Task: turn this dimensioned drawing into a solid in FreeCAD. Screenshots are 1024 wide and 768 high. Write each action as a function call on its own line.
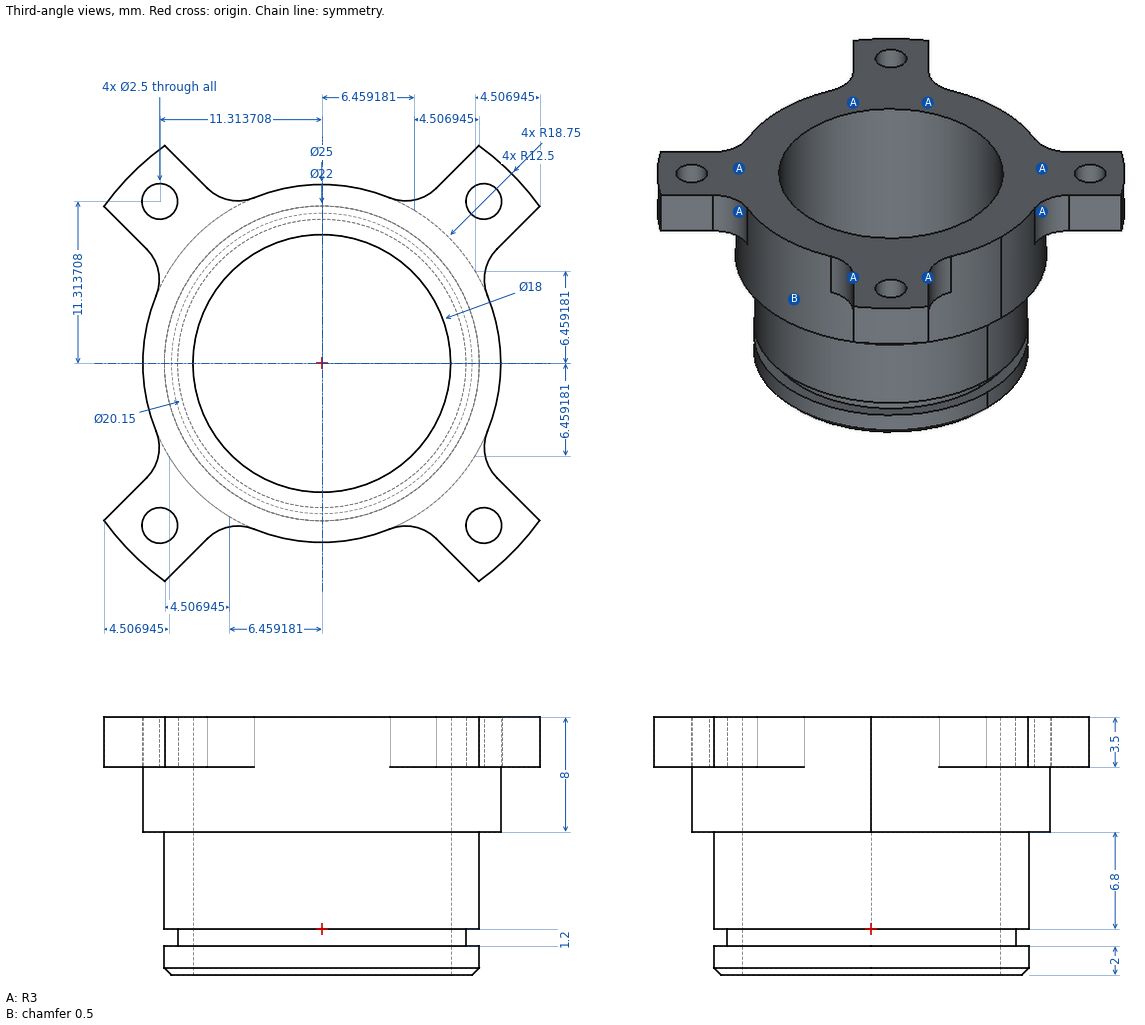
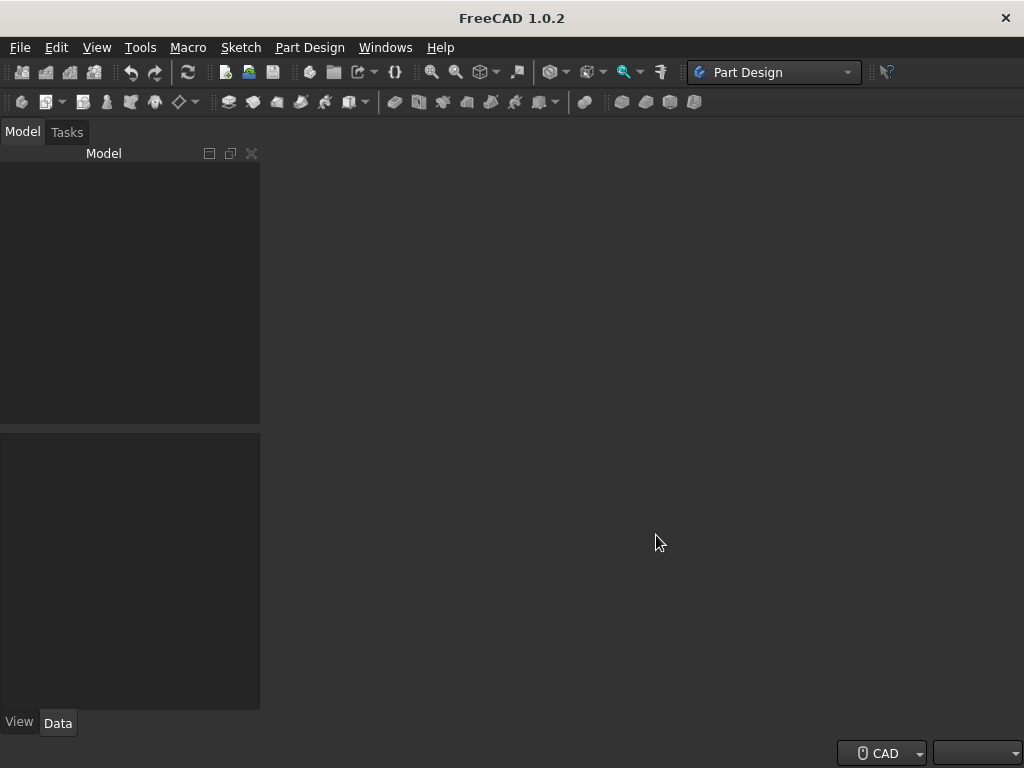
click(226, 72)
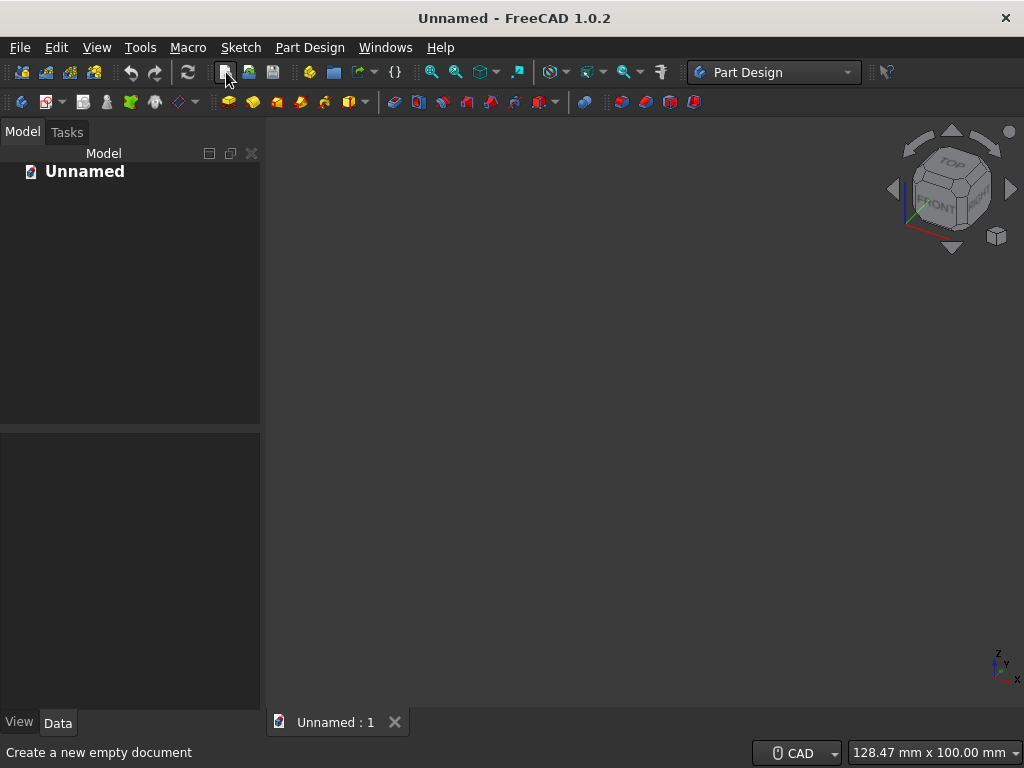
click(46, 102)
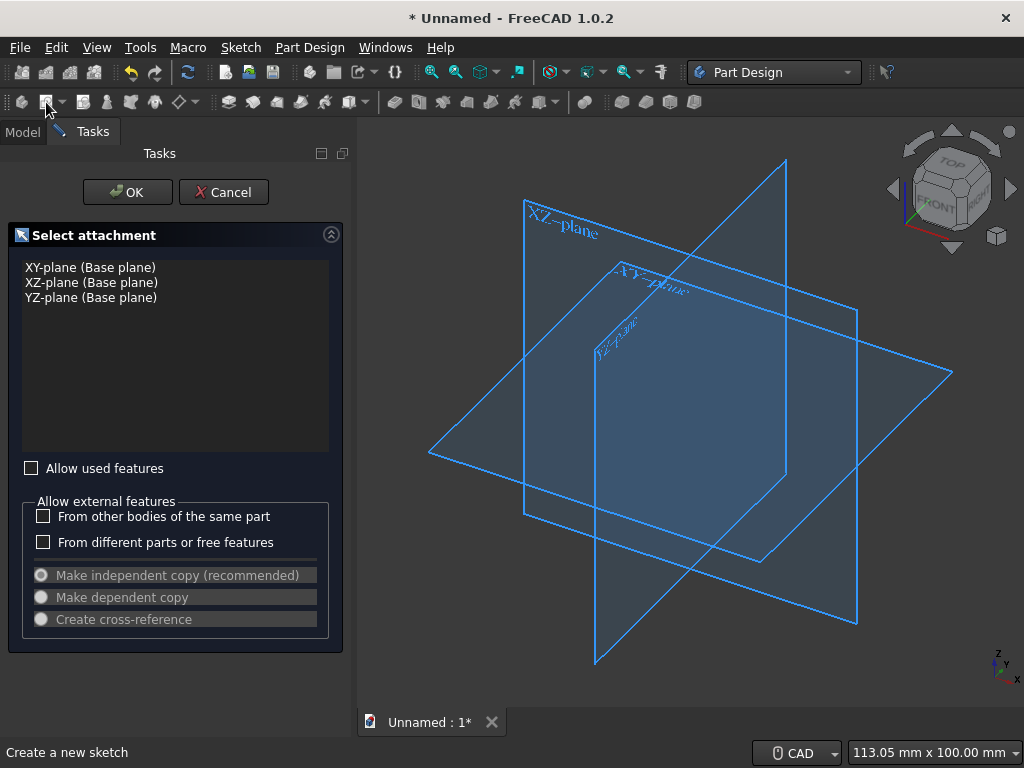
click(82, 268)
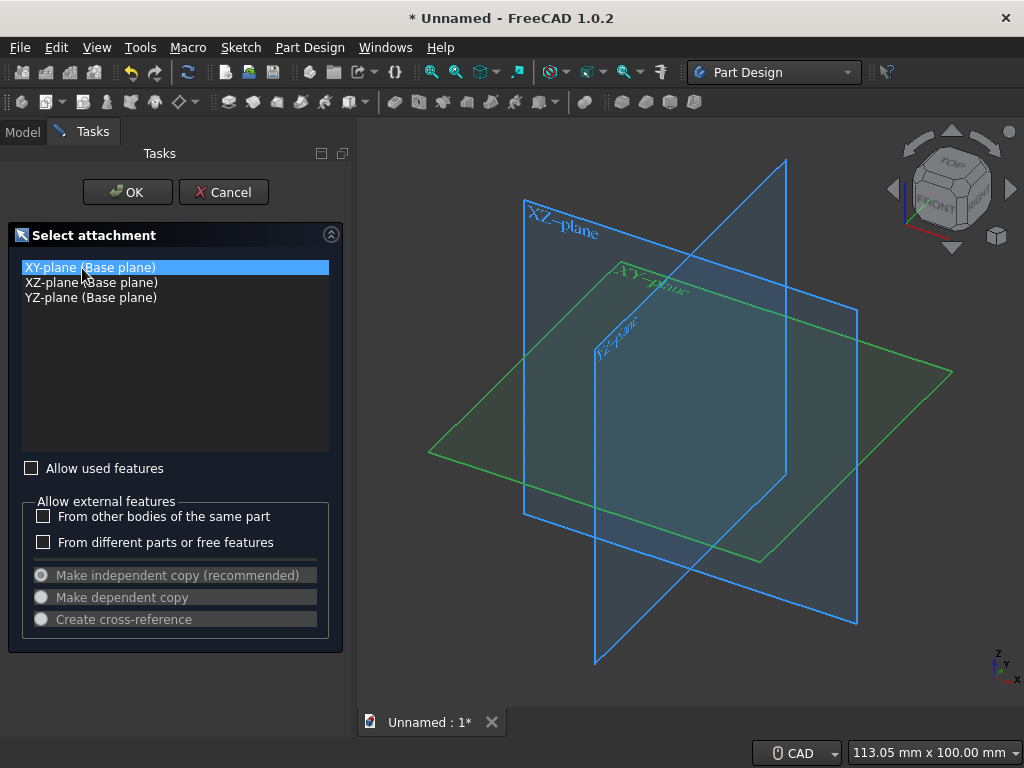
click(128, 192)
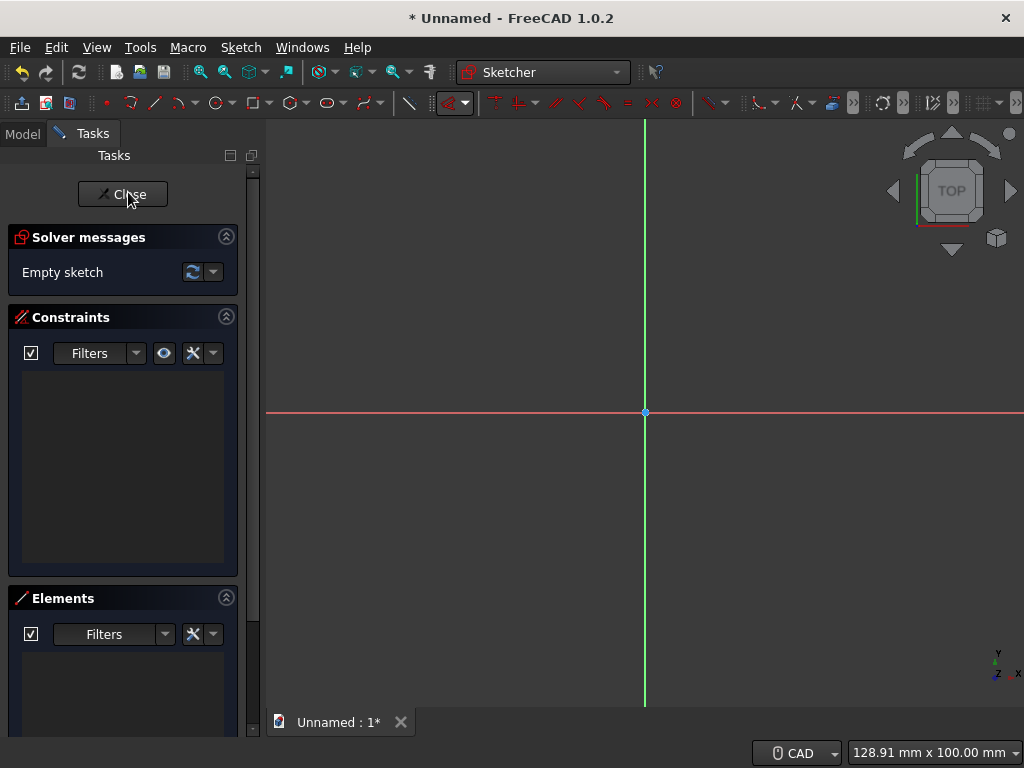
scroll(685, 413, up, 5)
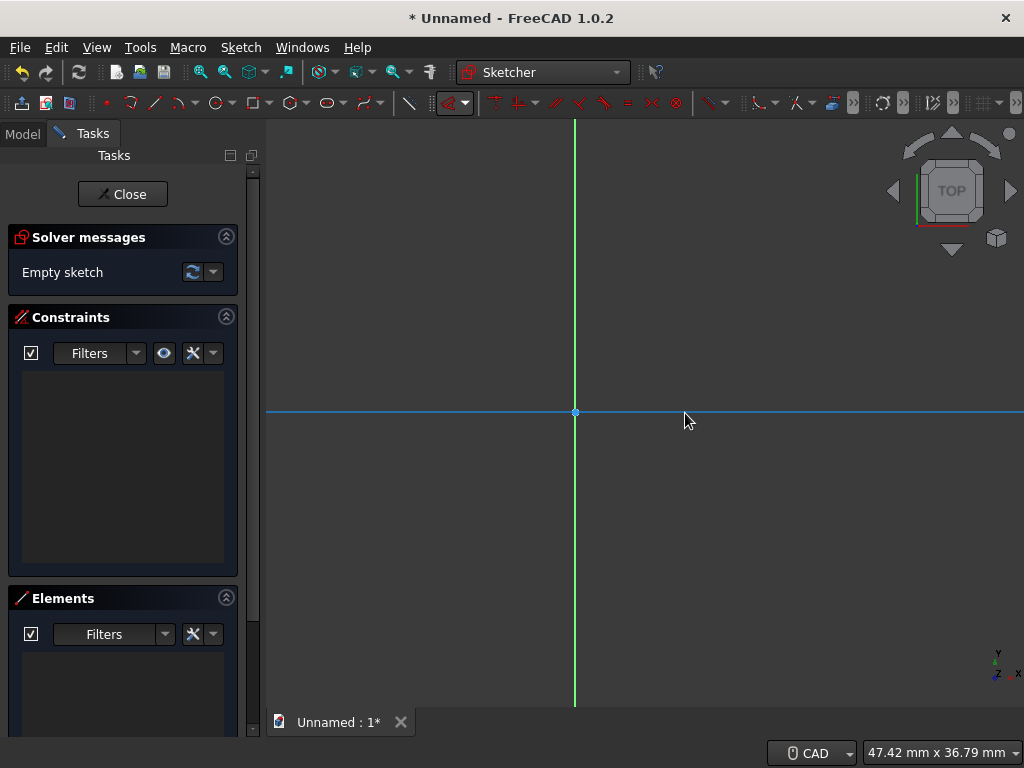
click(216, 104)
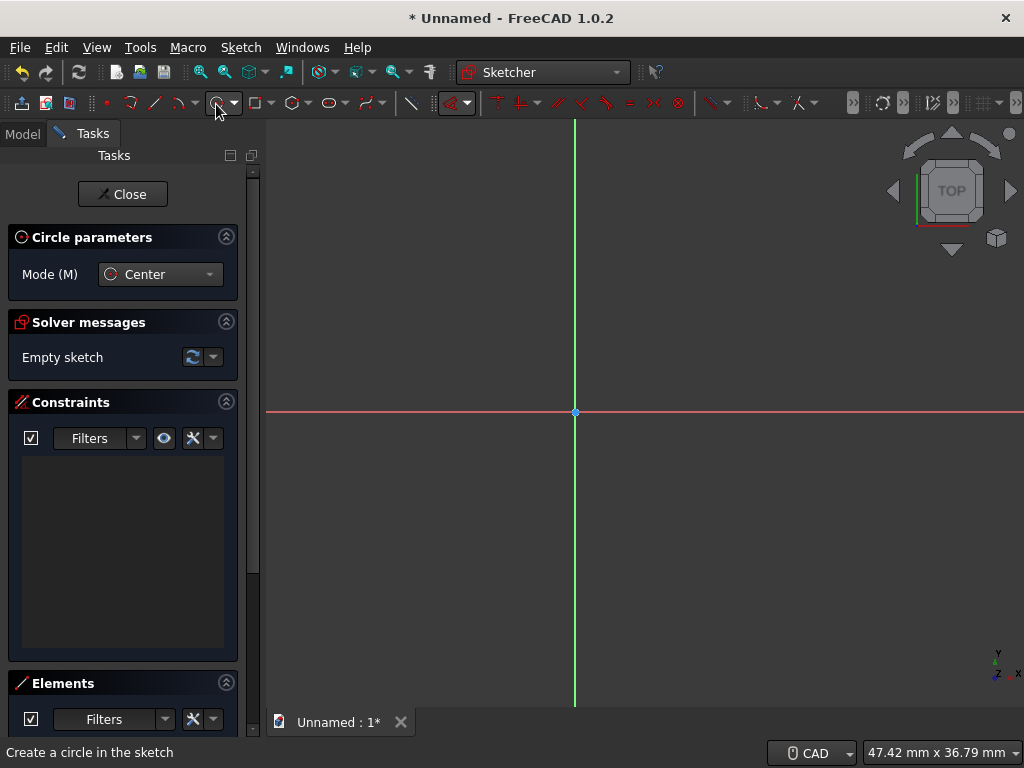
click(575, 412)
click(700, 288)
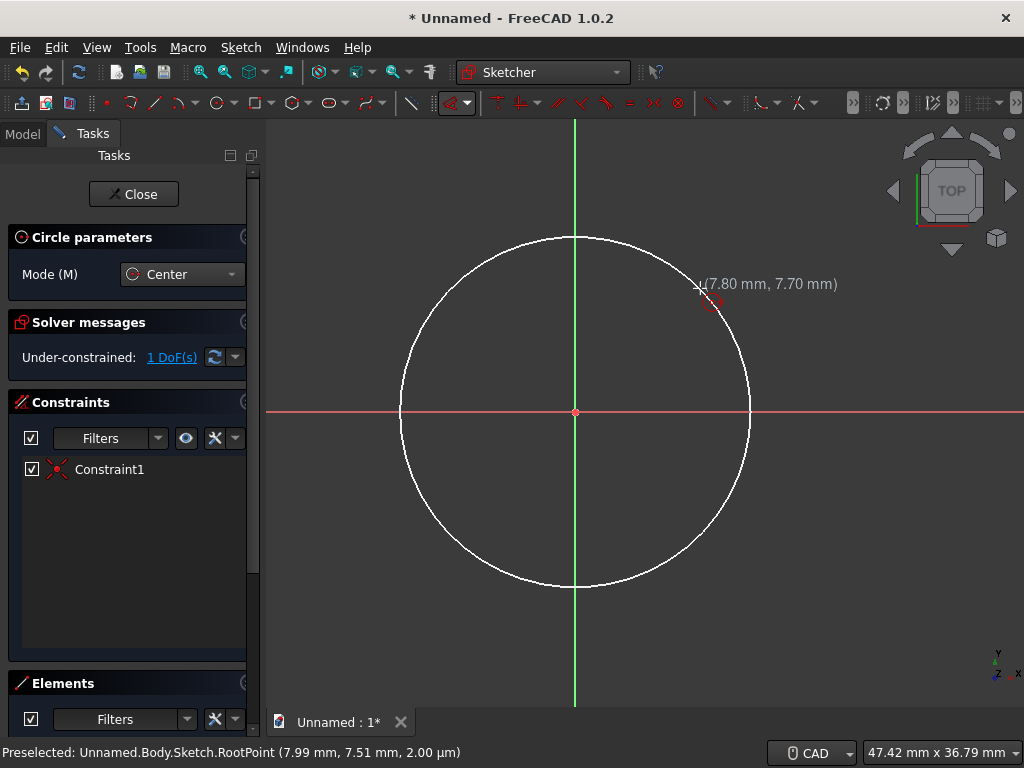
click(575, 412)
click(677, 310)
key(Escape)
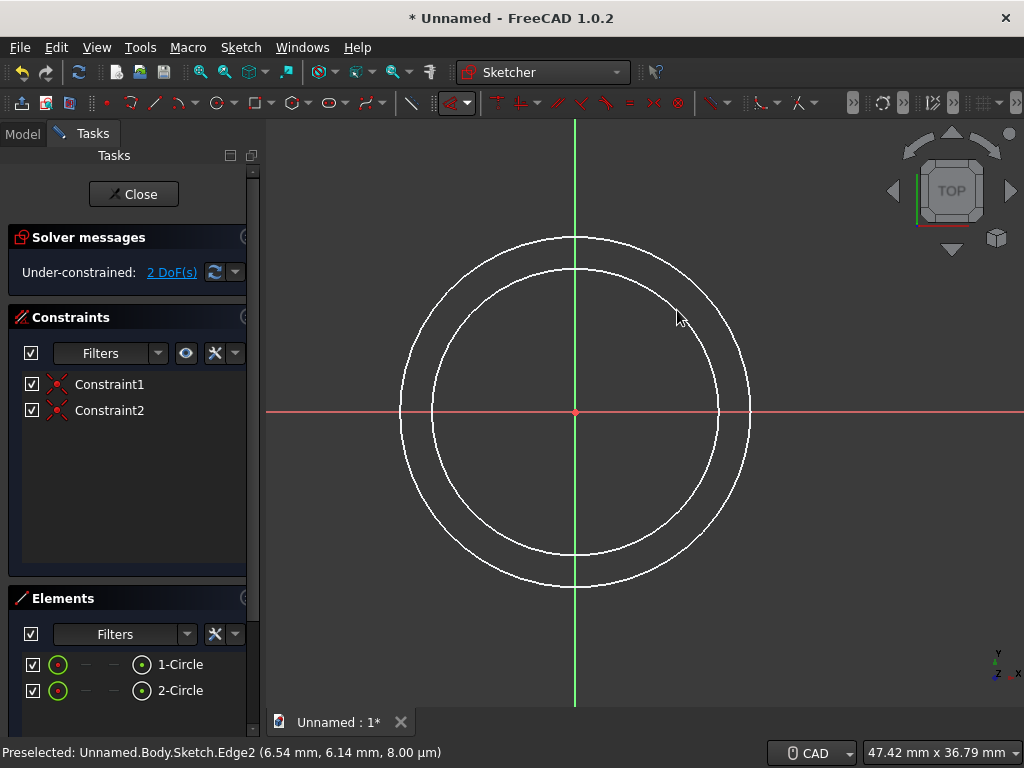
click(450, 104)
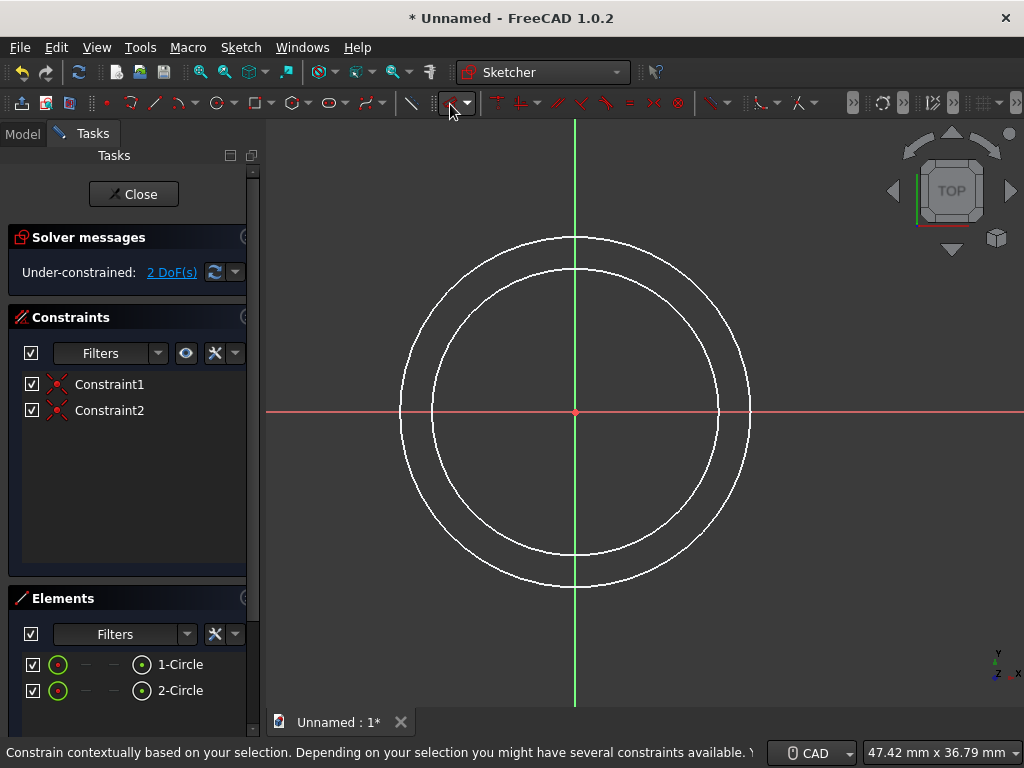
click(699, 288)
click(722, 265)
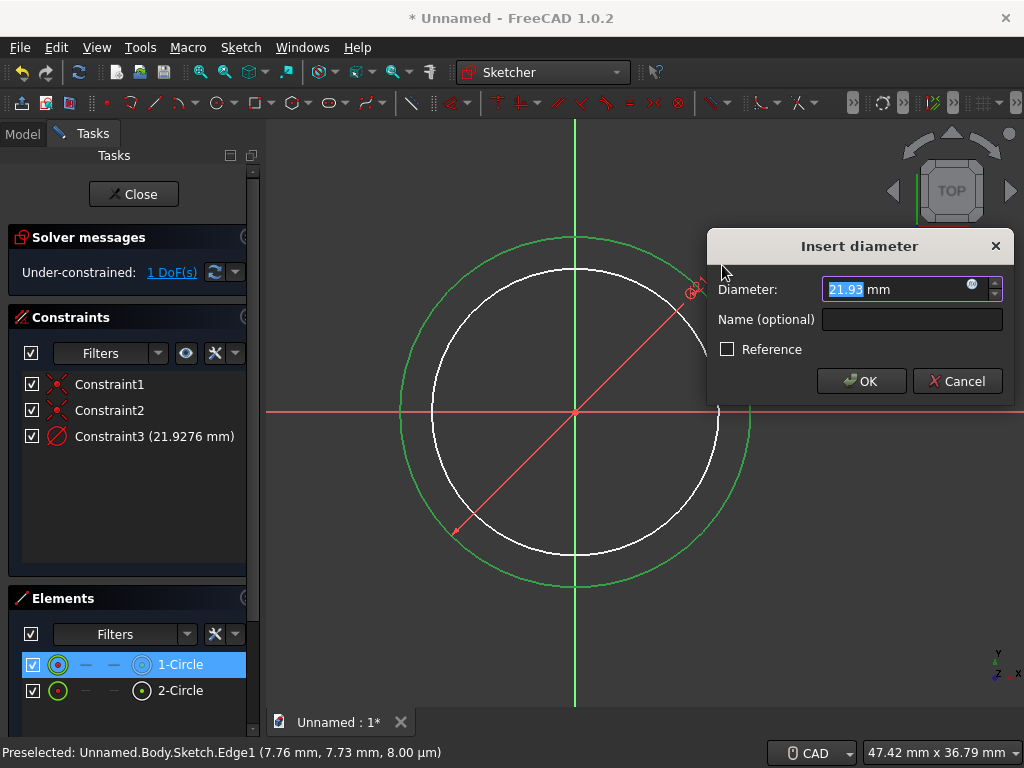
text(22)
key(Return)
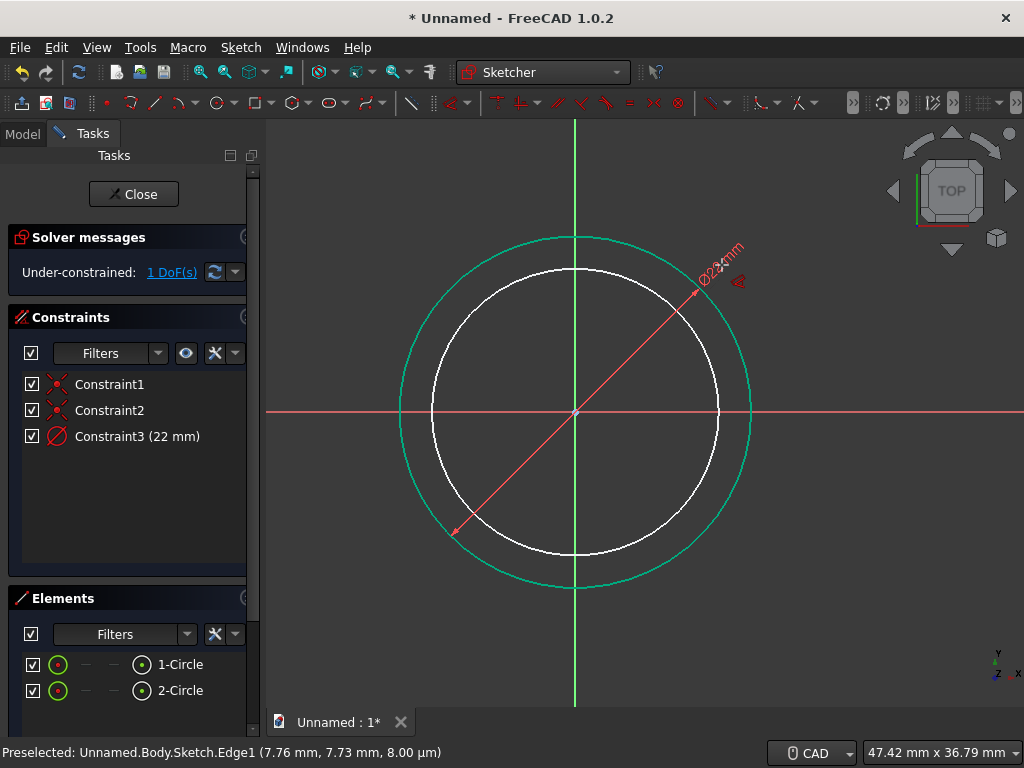
click(676, 310)
click(765, 355)